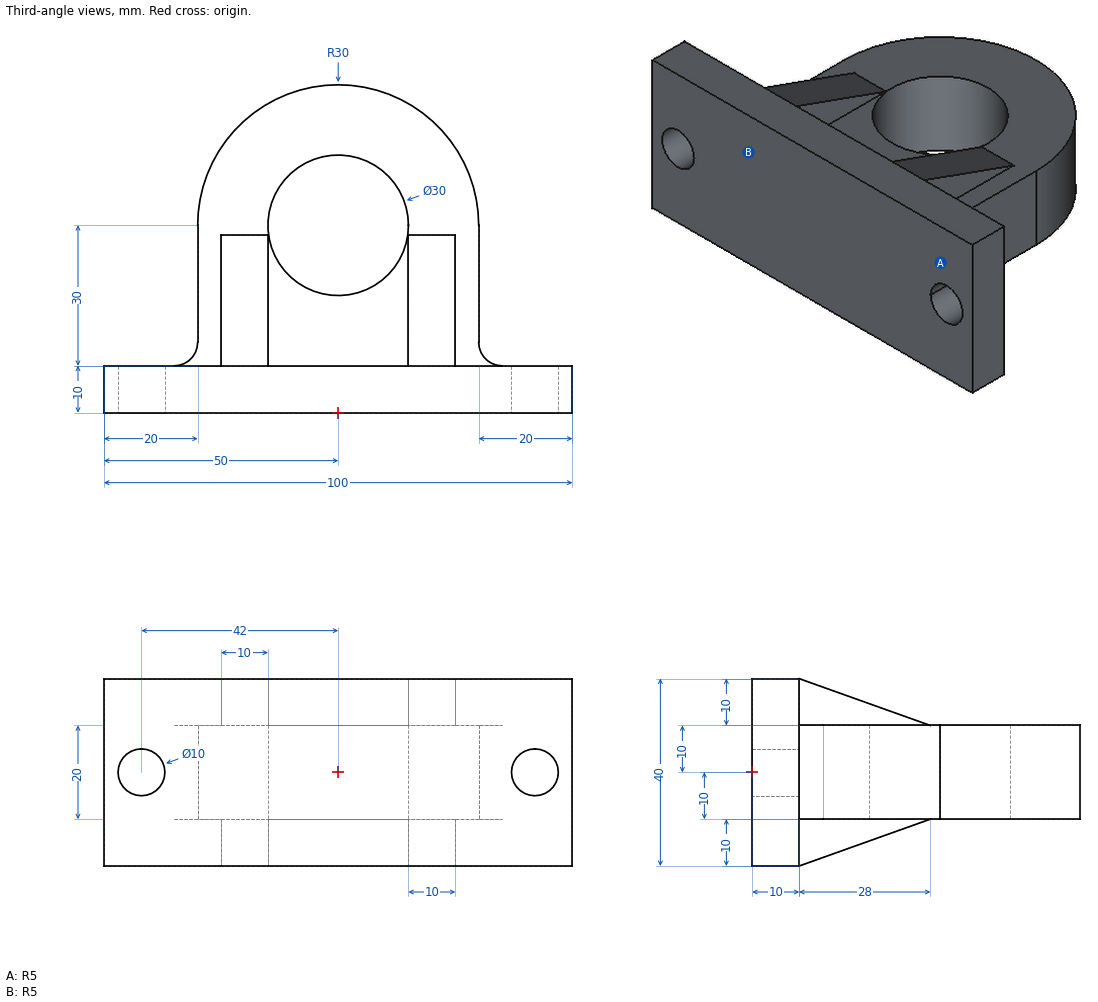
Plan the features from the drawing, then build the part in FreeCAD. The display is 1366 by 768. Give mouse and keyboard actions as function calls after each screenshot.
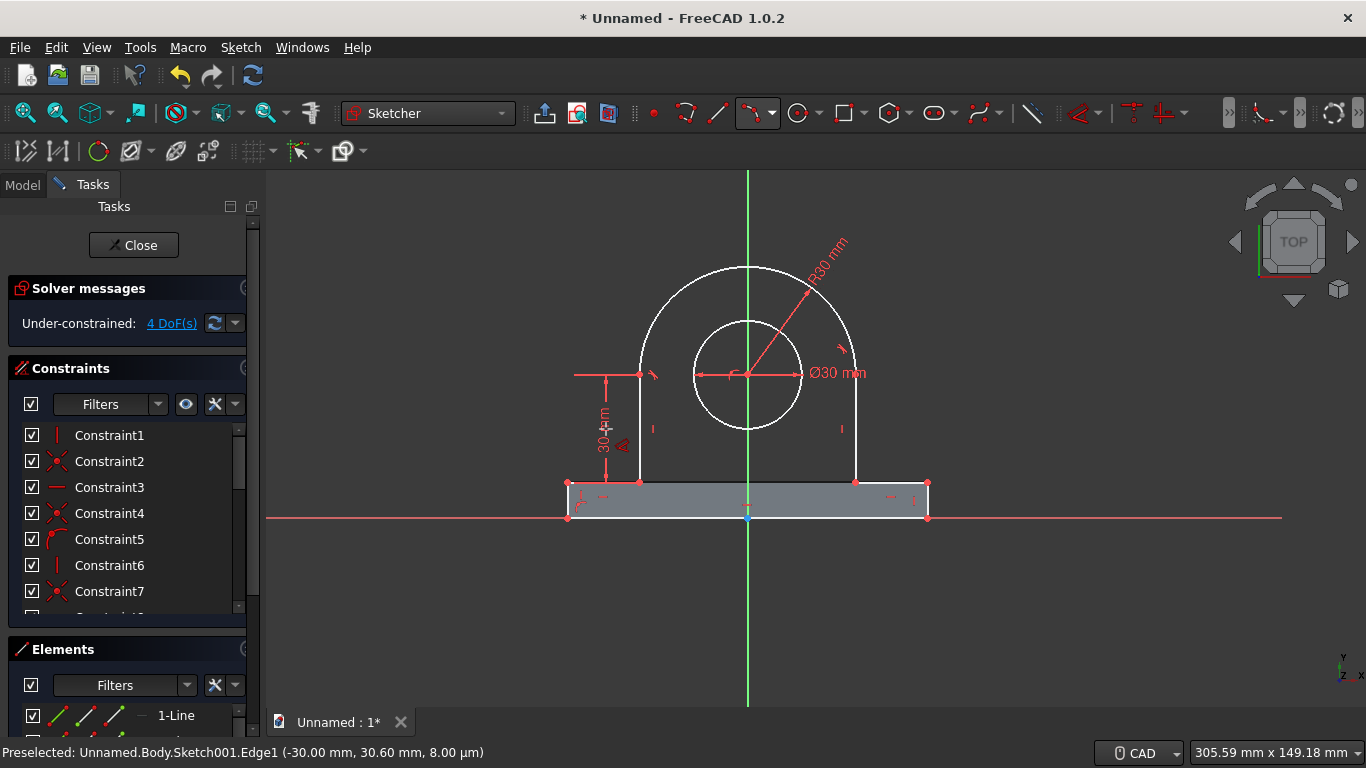
click(618, 483)
click(604, 449)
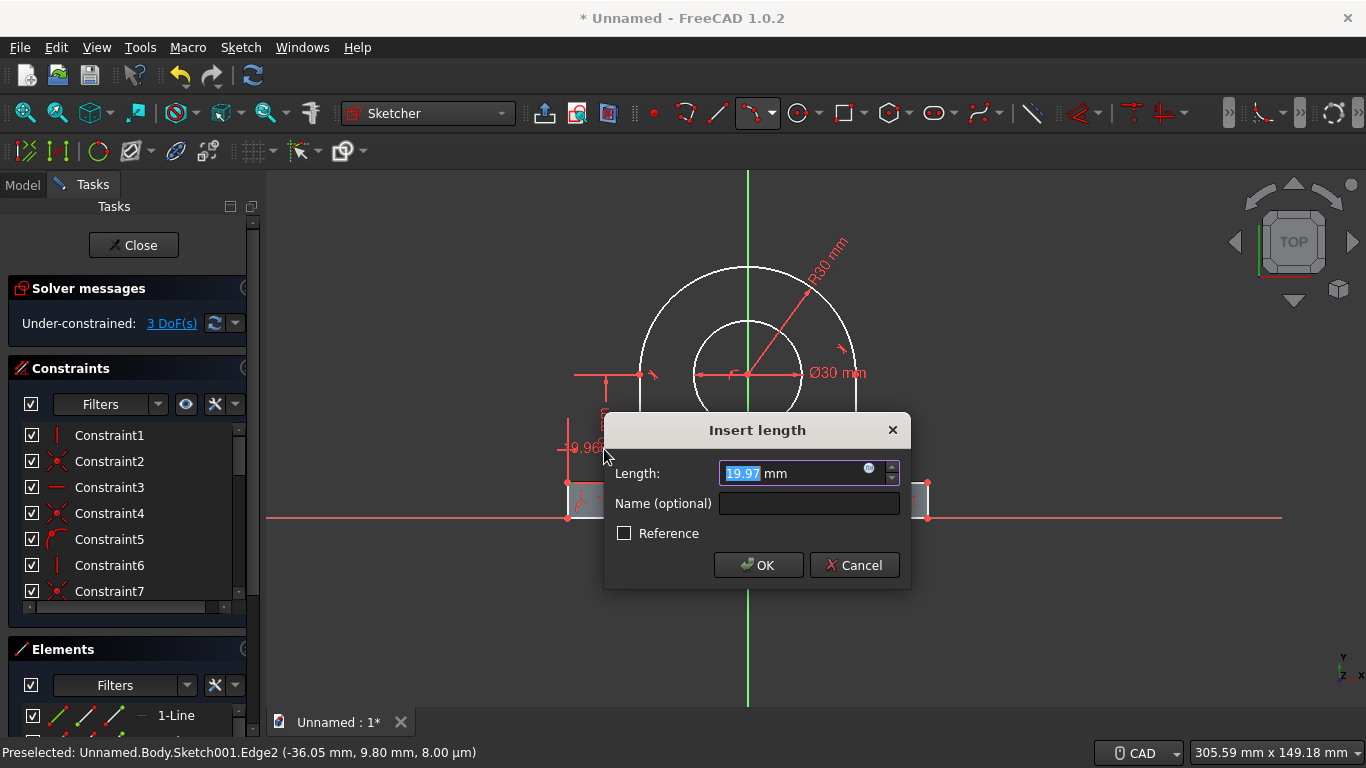
text(20)
key(Return)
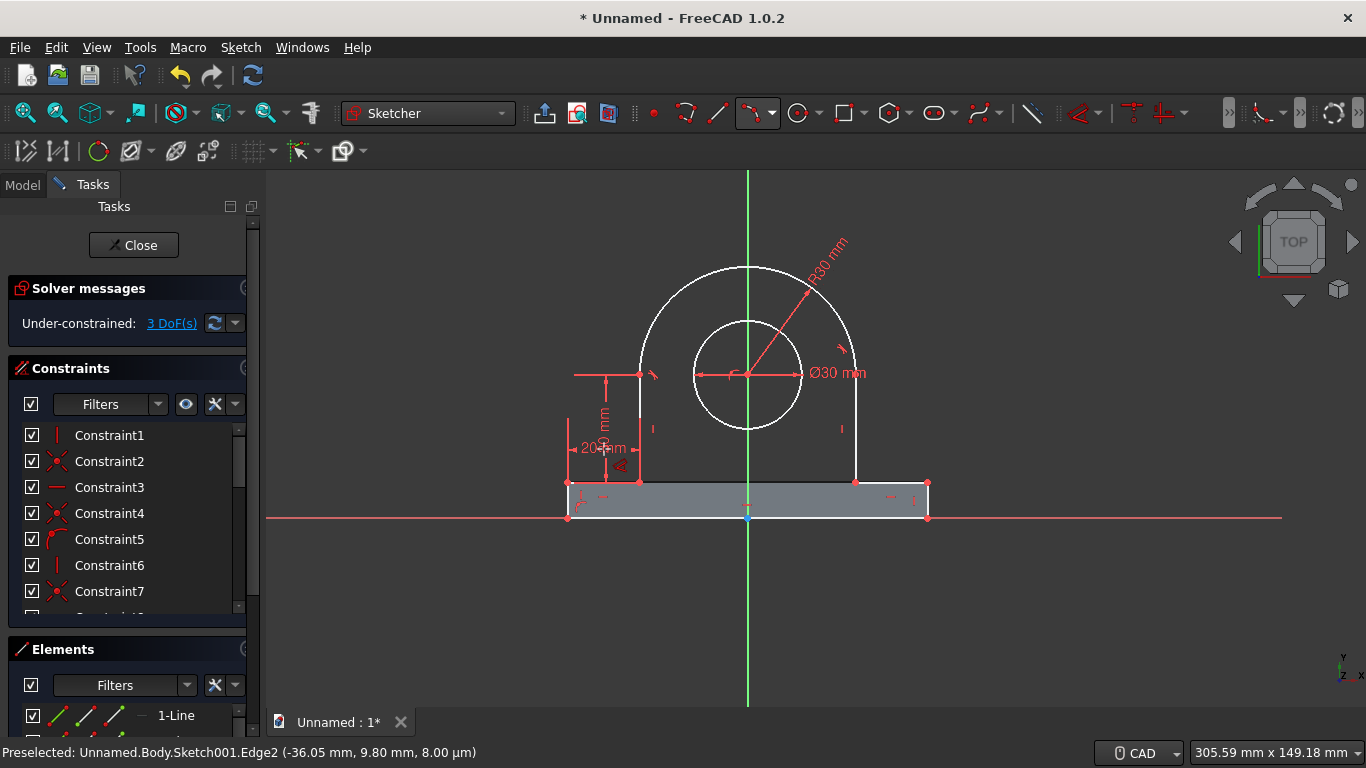
scroll(568, 493, up, 2)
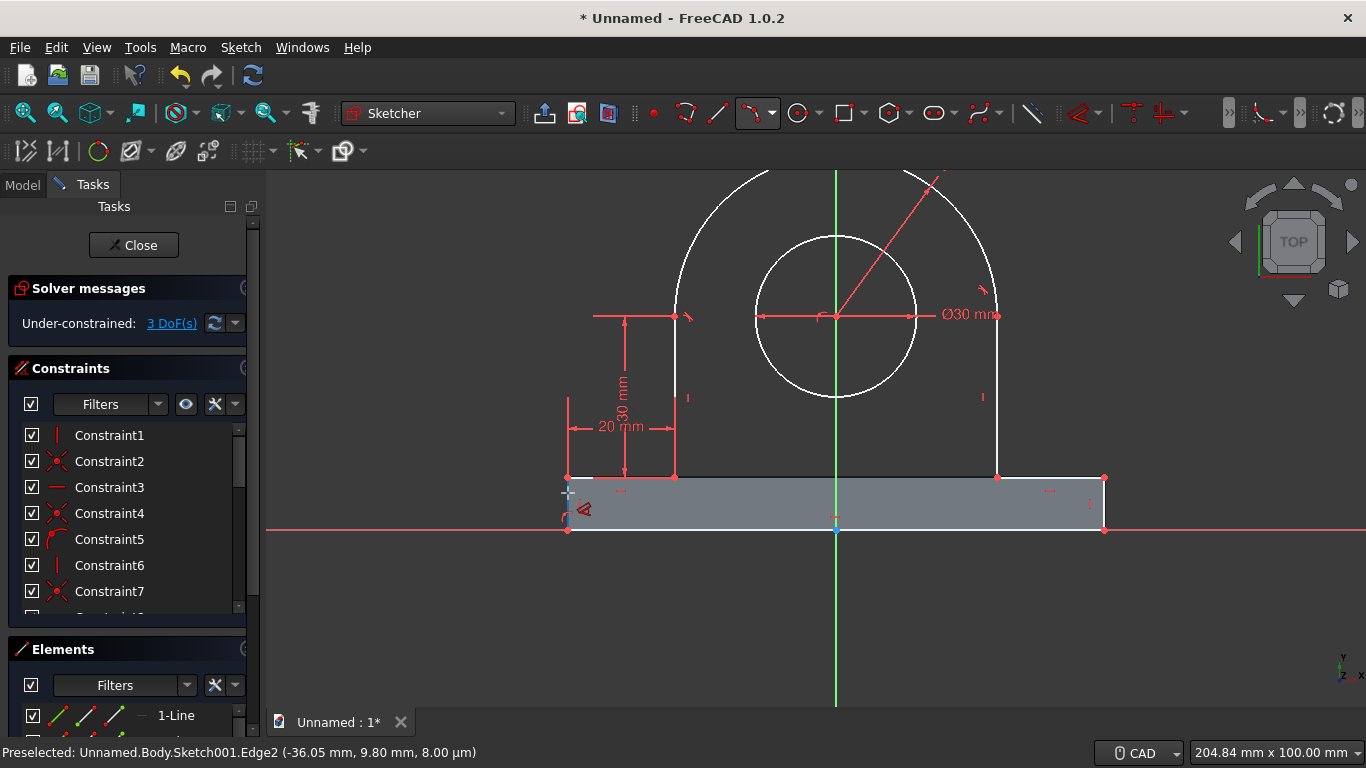
click(568, 493)
click(534, 504)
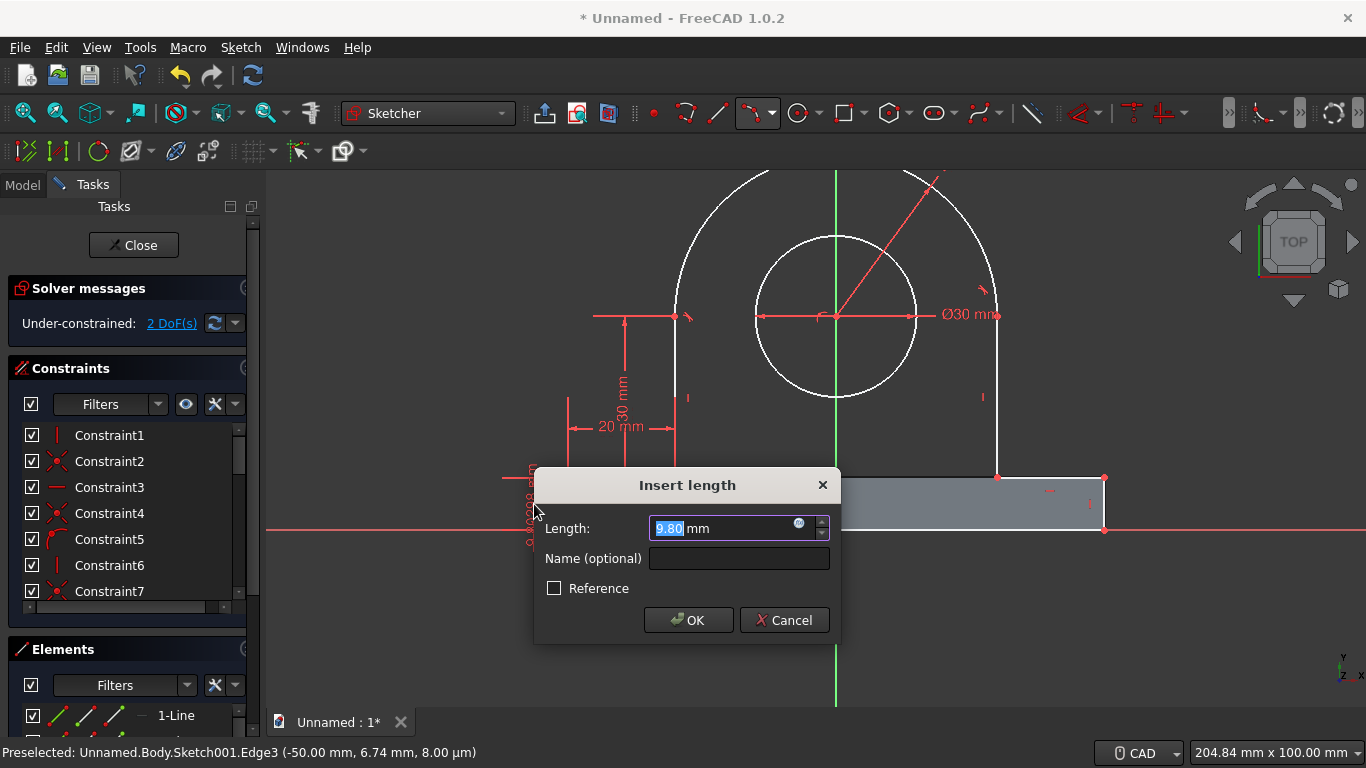
text(10)
key(Return)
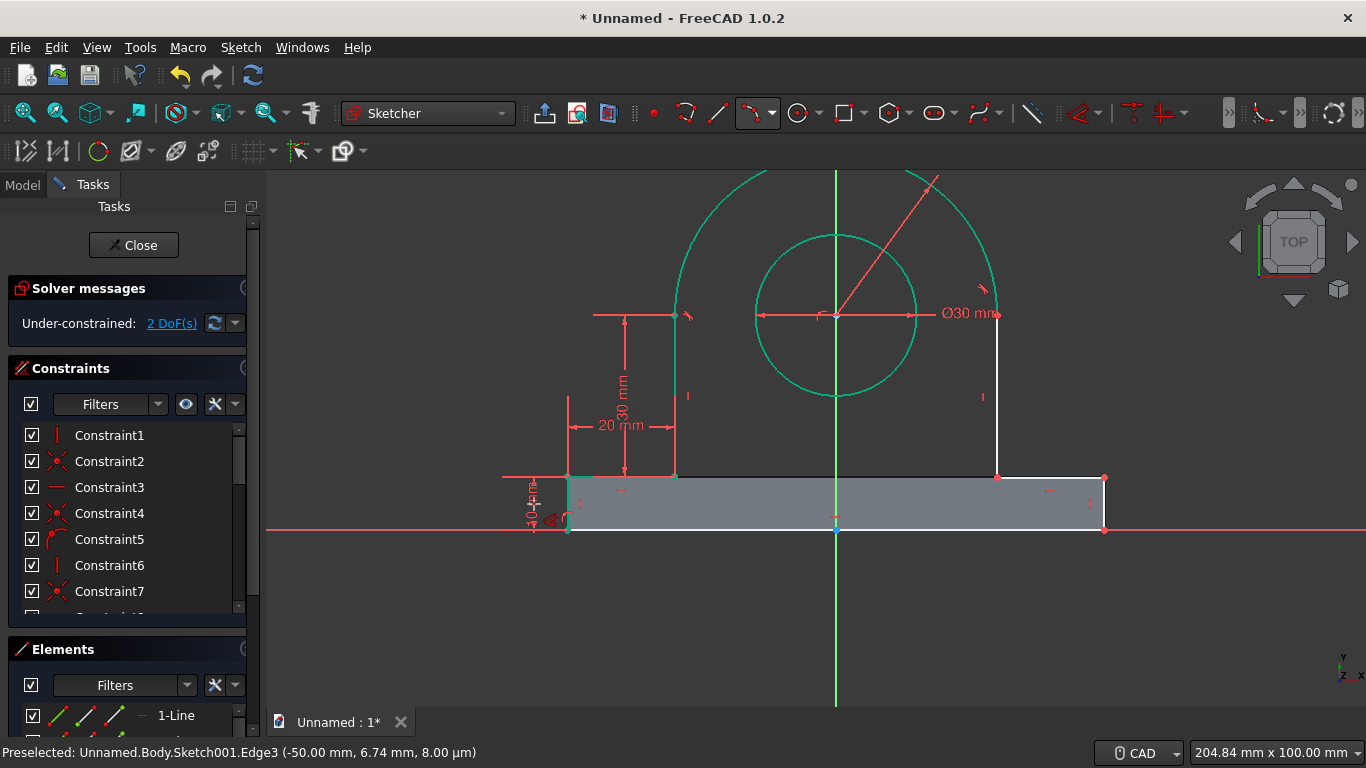
click(1104, 514)
click(1138, 504)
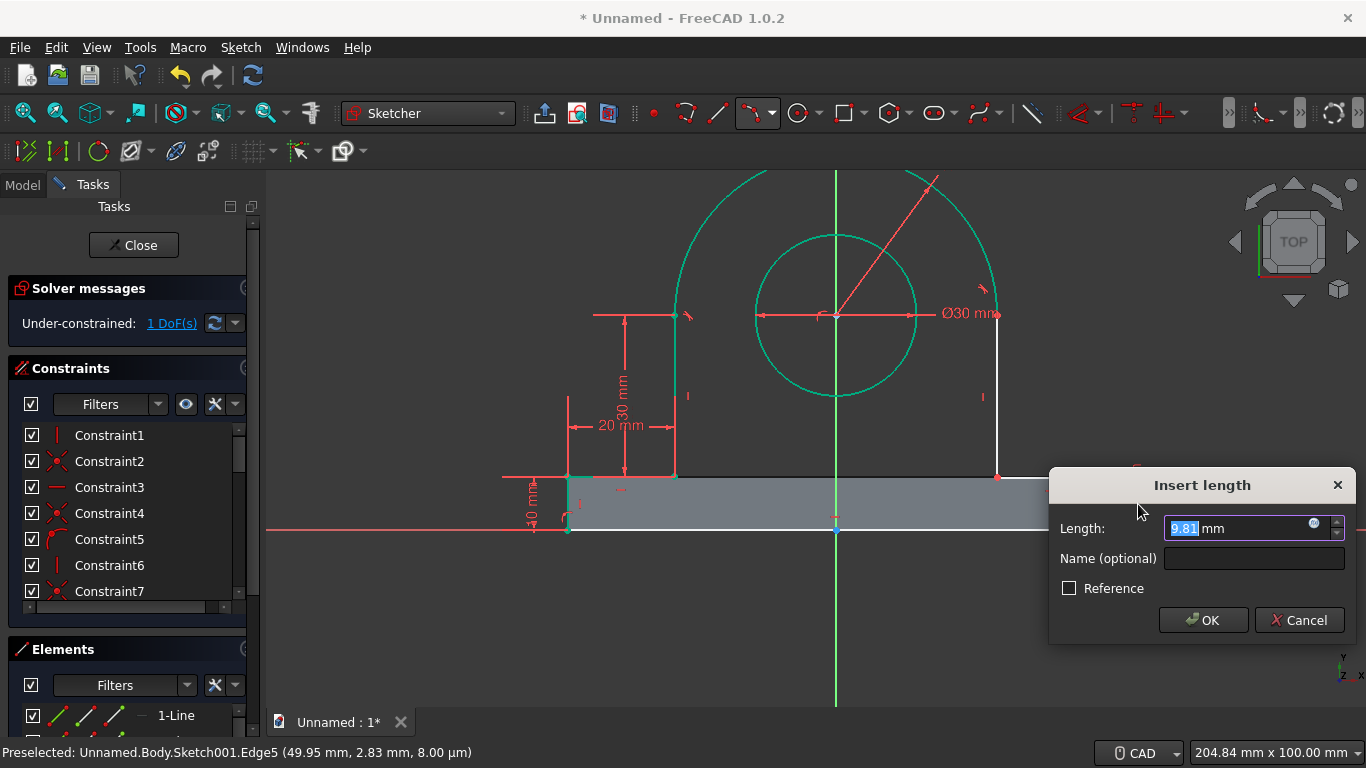
text(10)
key(Return)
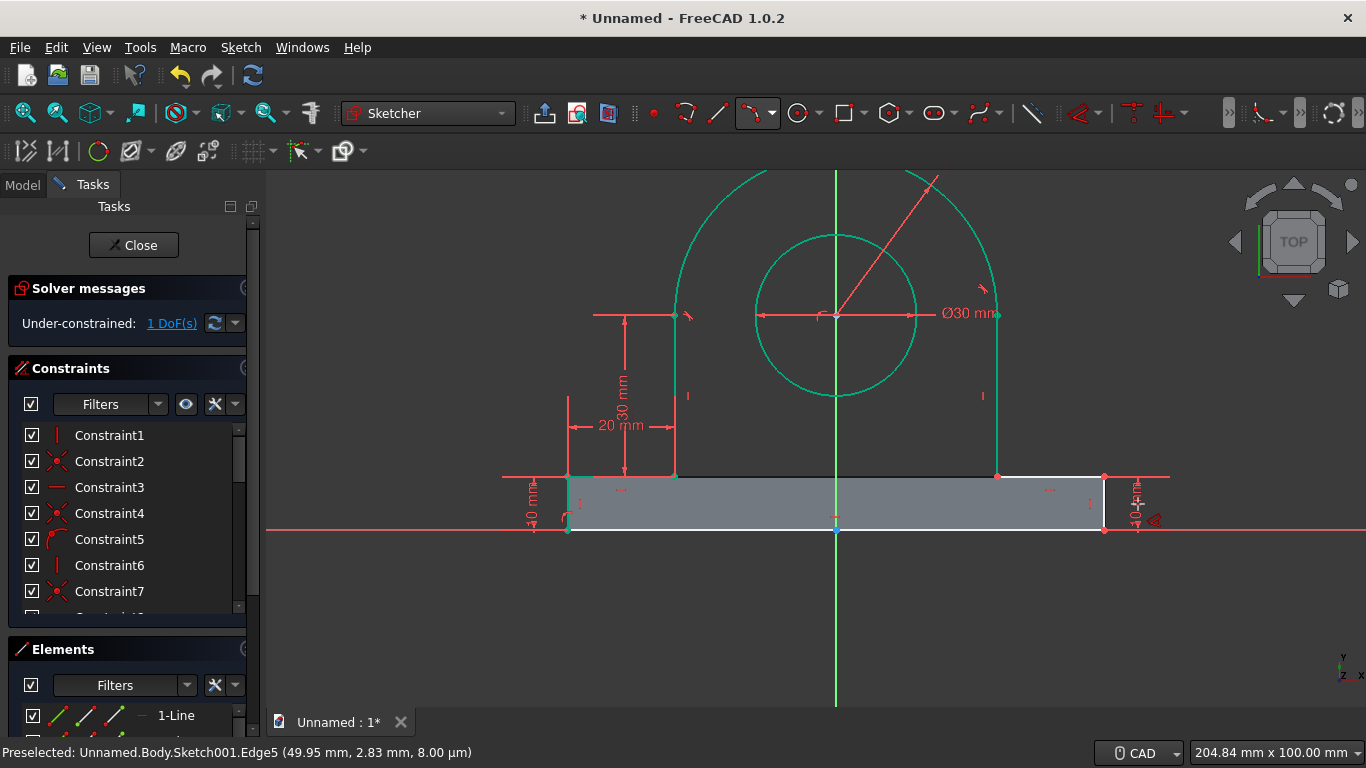
click(1072, 476)
click(1051, 510)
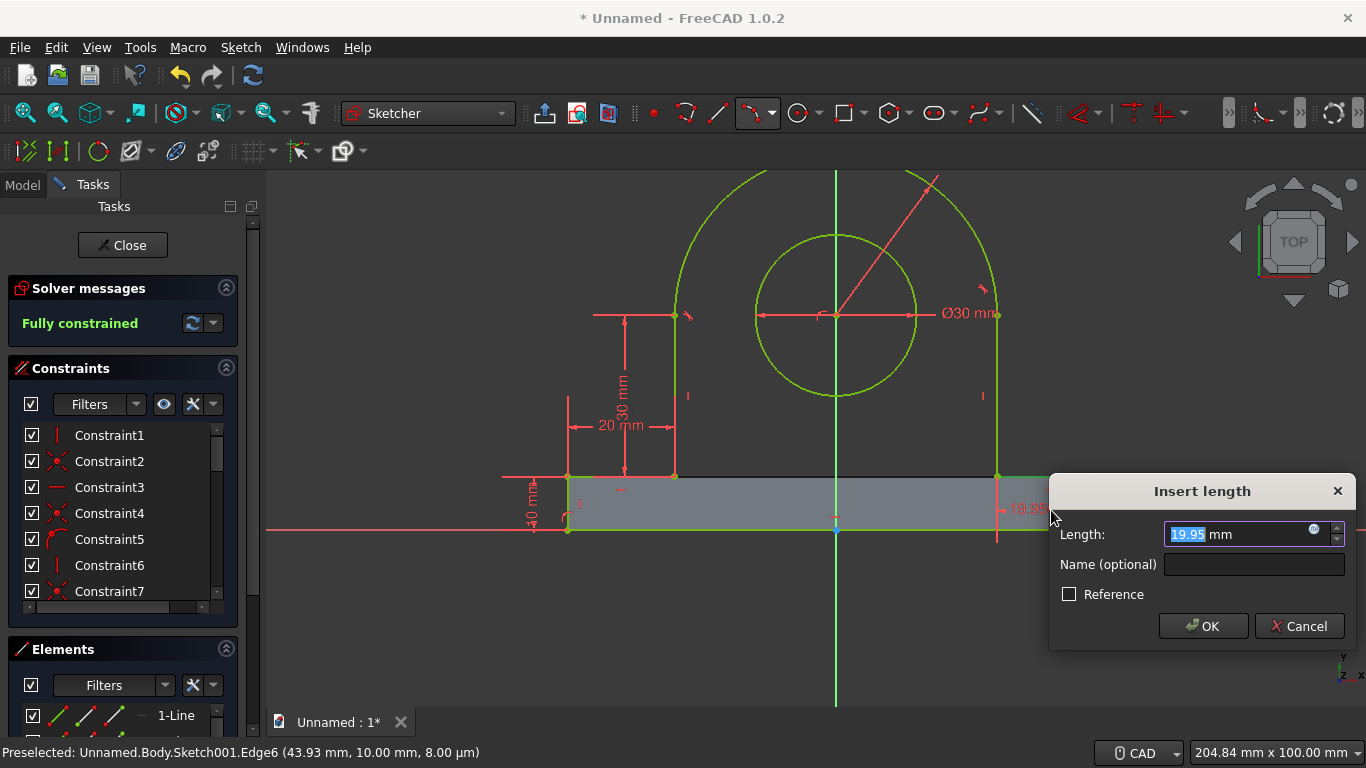
text(20)
key(Return)
key(Escape)